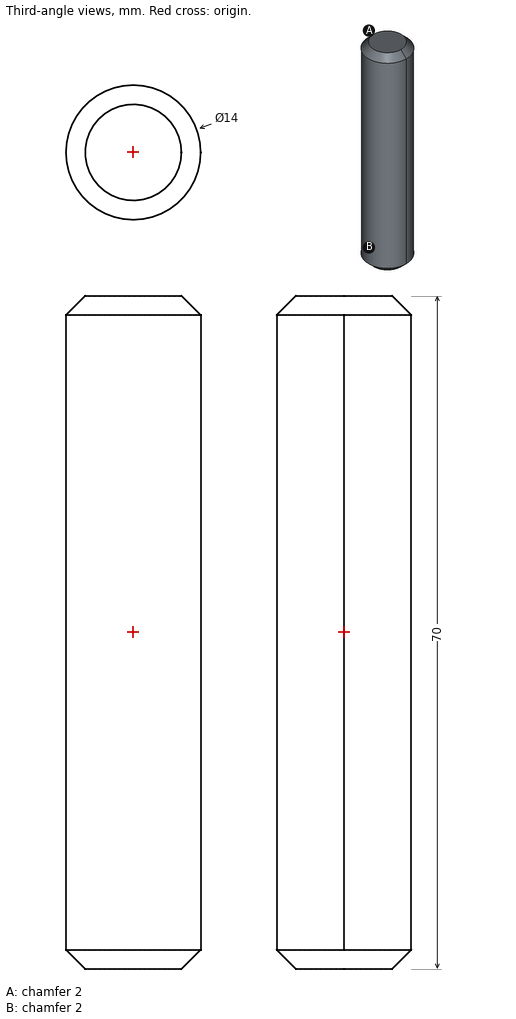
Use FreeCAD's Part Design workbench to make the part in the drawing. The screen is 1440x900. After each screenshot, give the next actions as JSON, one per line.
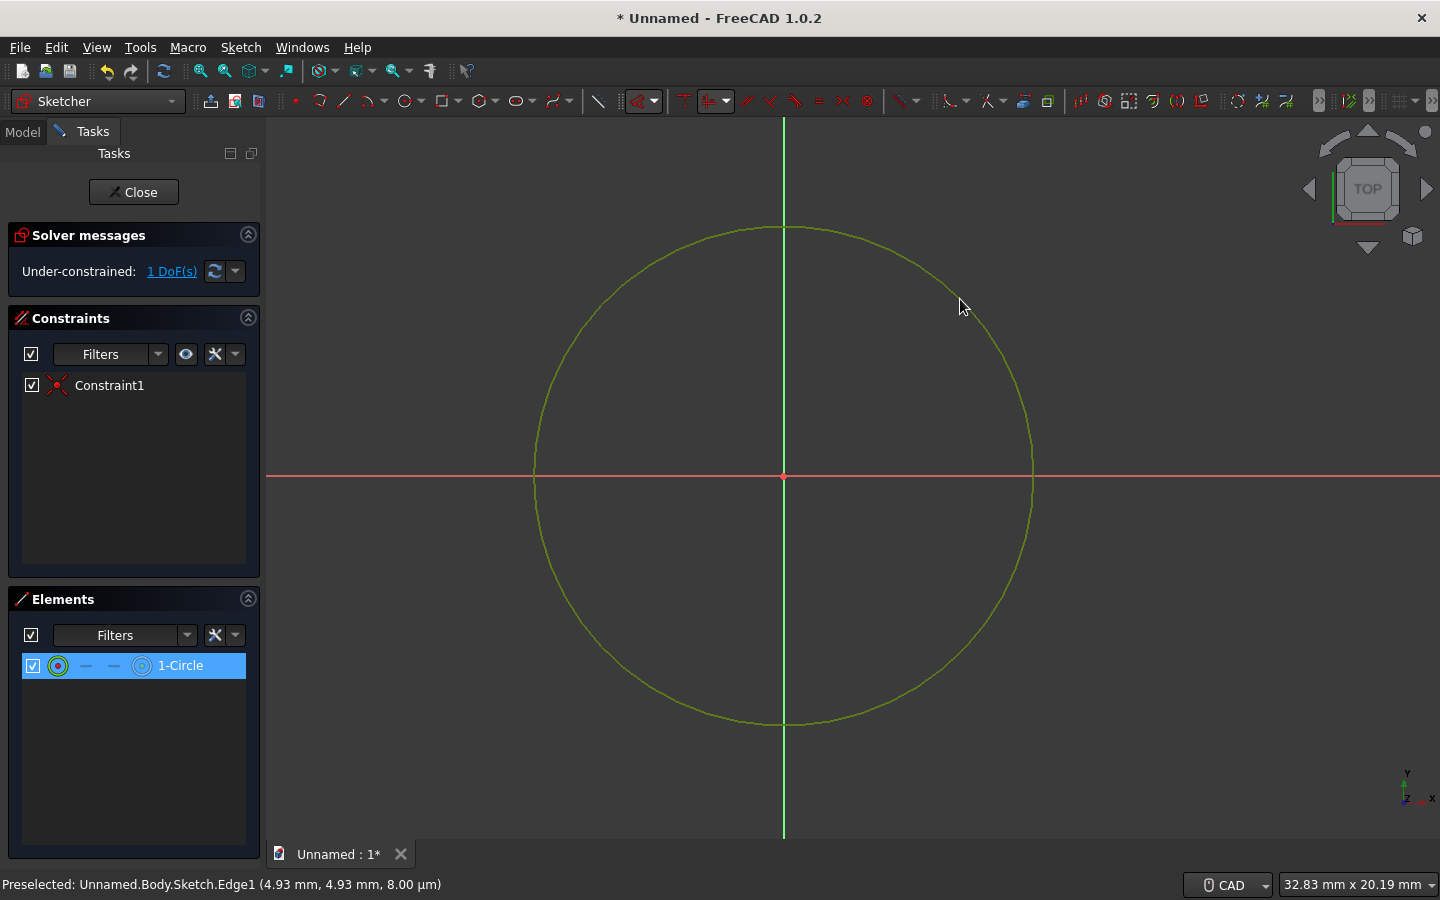
{"action": "key", "text": "k o"}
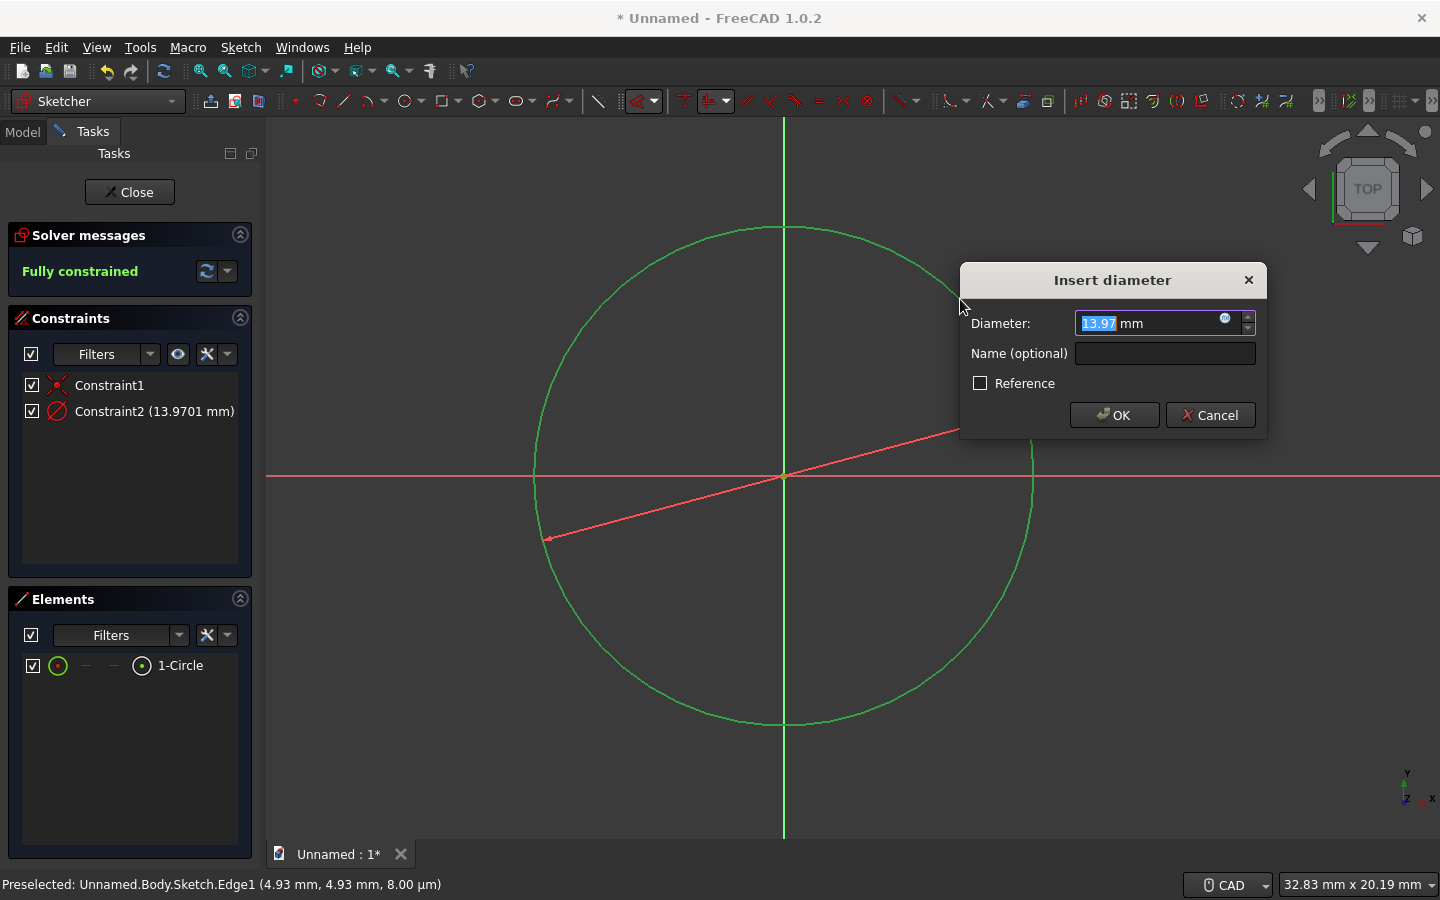
{"action": "type", "text": "14"}
{"action": "key", "text": "Return"}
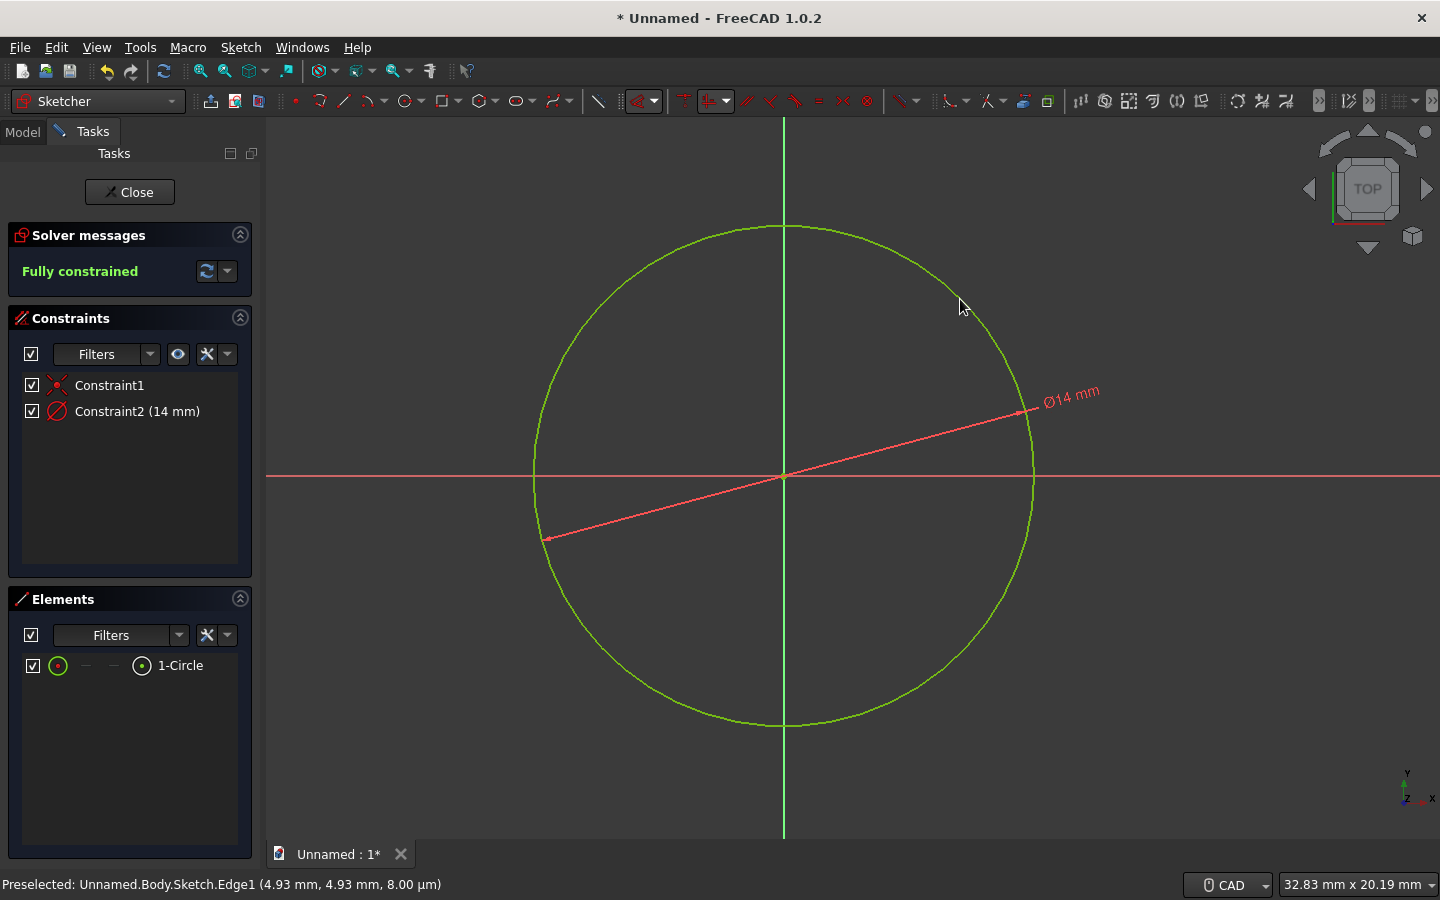
{"action": "left_click", "coordinate": [130, 192]}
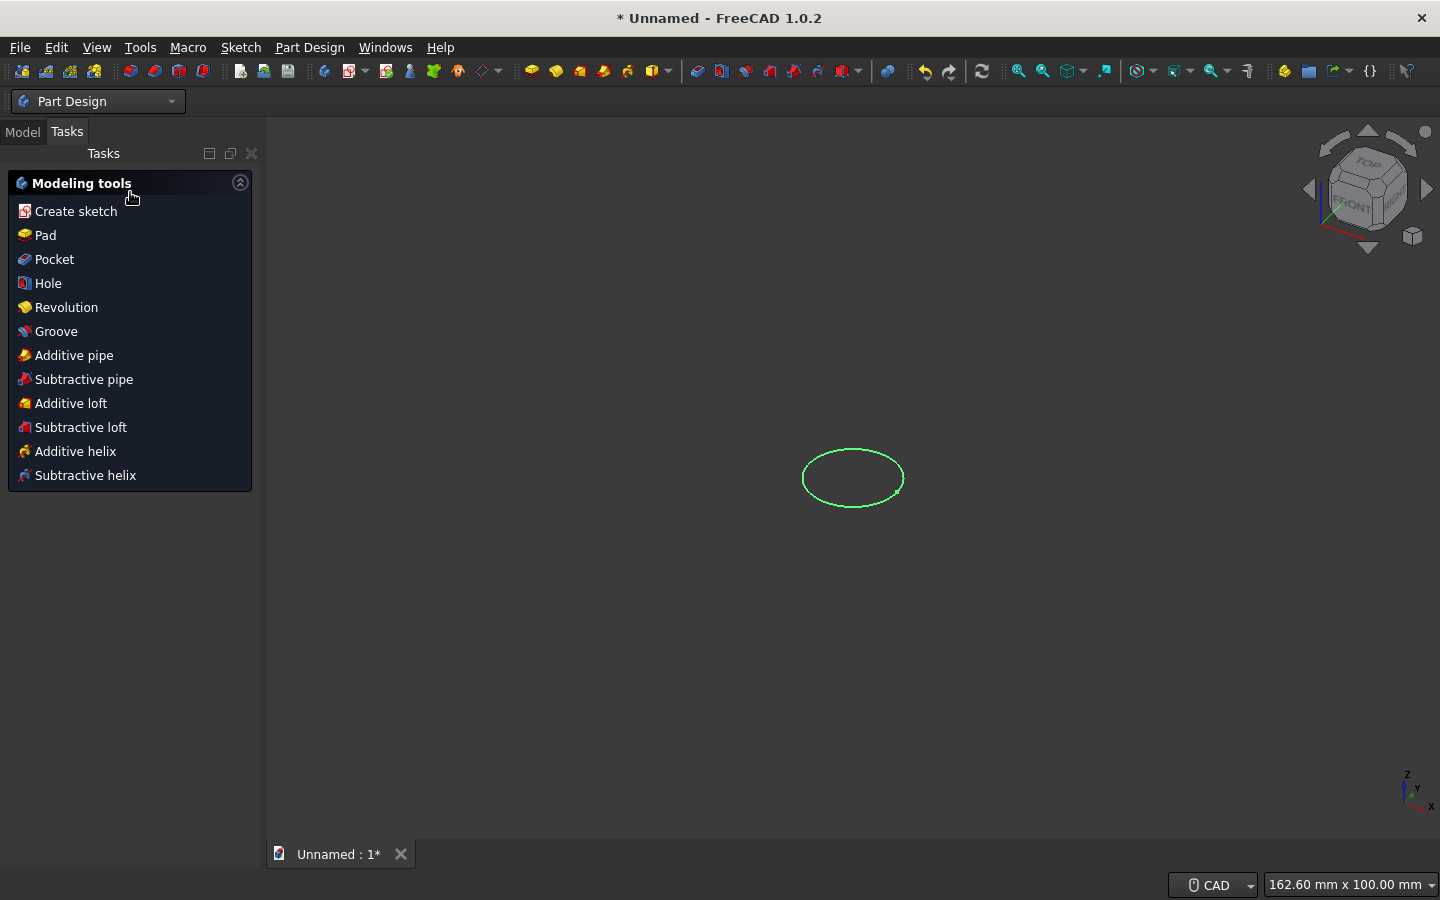
{"action": "left_click", "coordinate": [532, 72]}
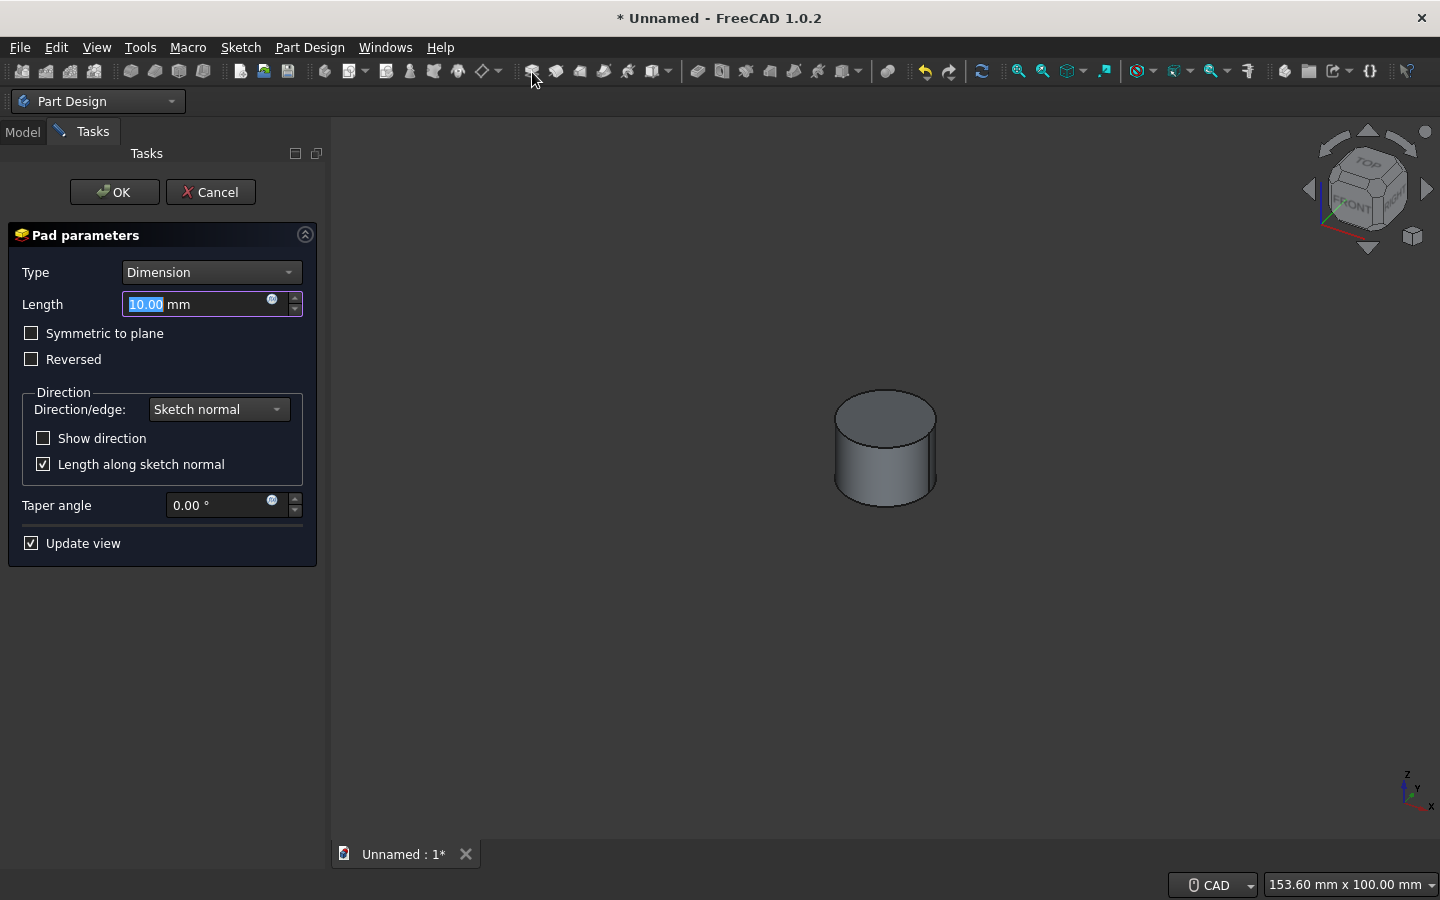
{"action": "type", "text": "70"}
{"action": "key", "text": "Tab"}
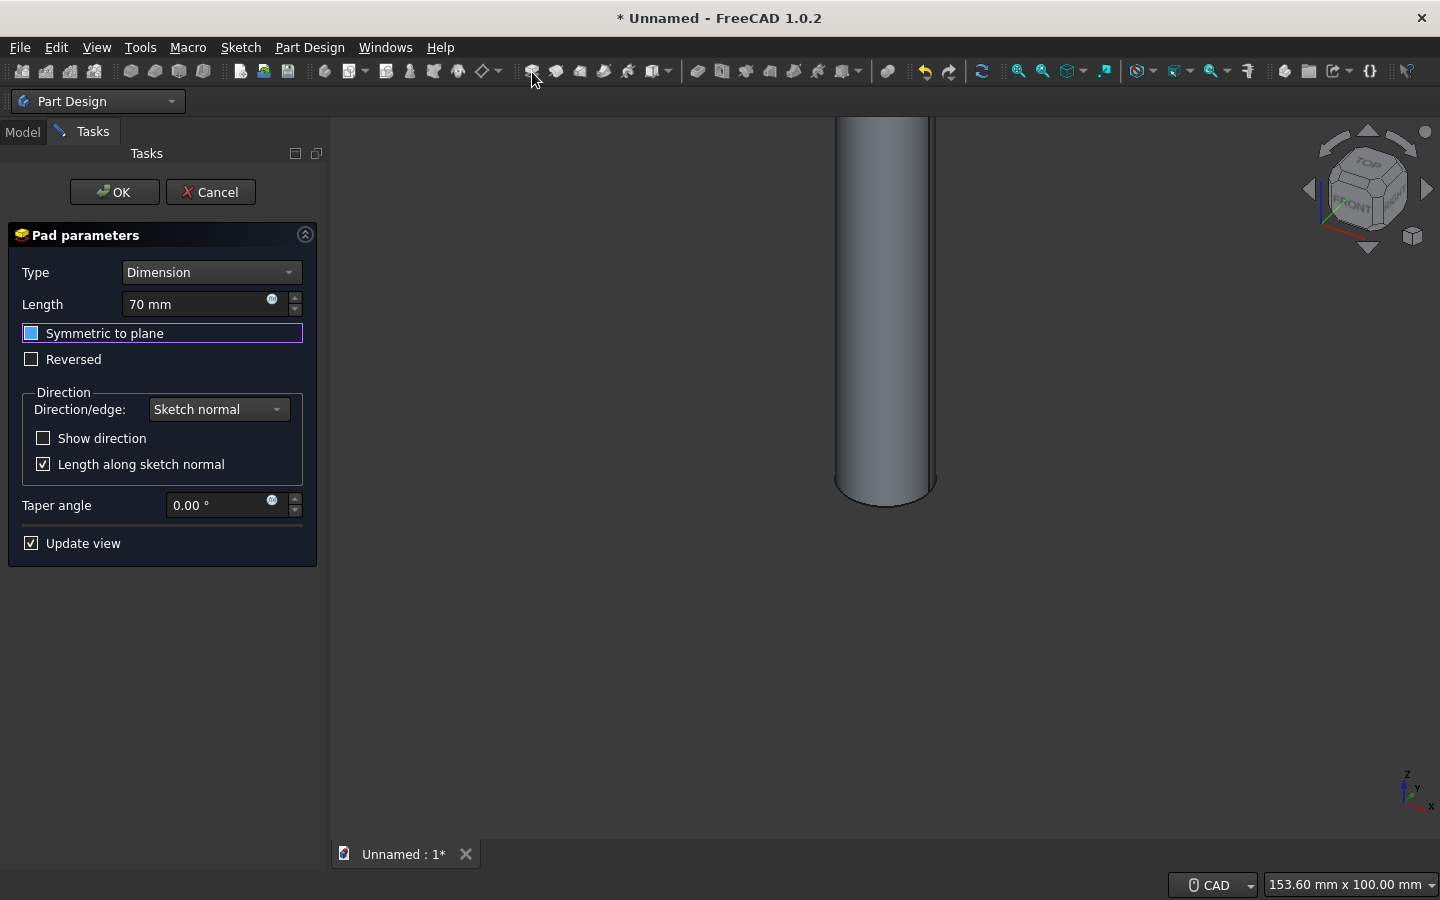
{"action": "left_click", "coordinate": [30, 333]}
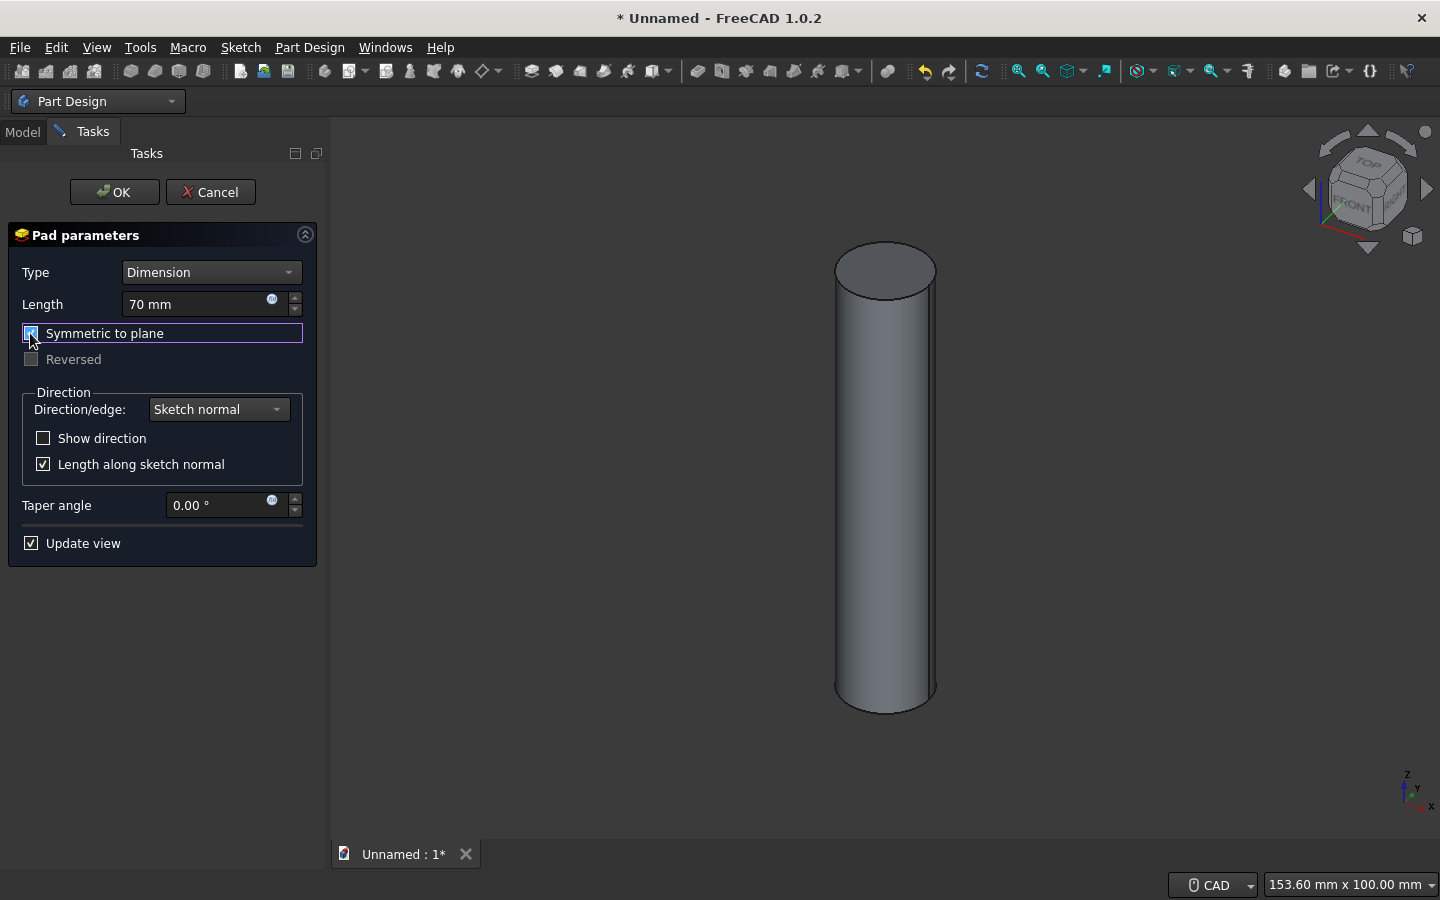
{"action": "left_click", "coordinate": [115, 192]}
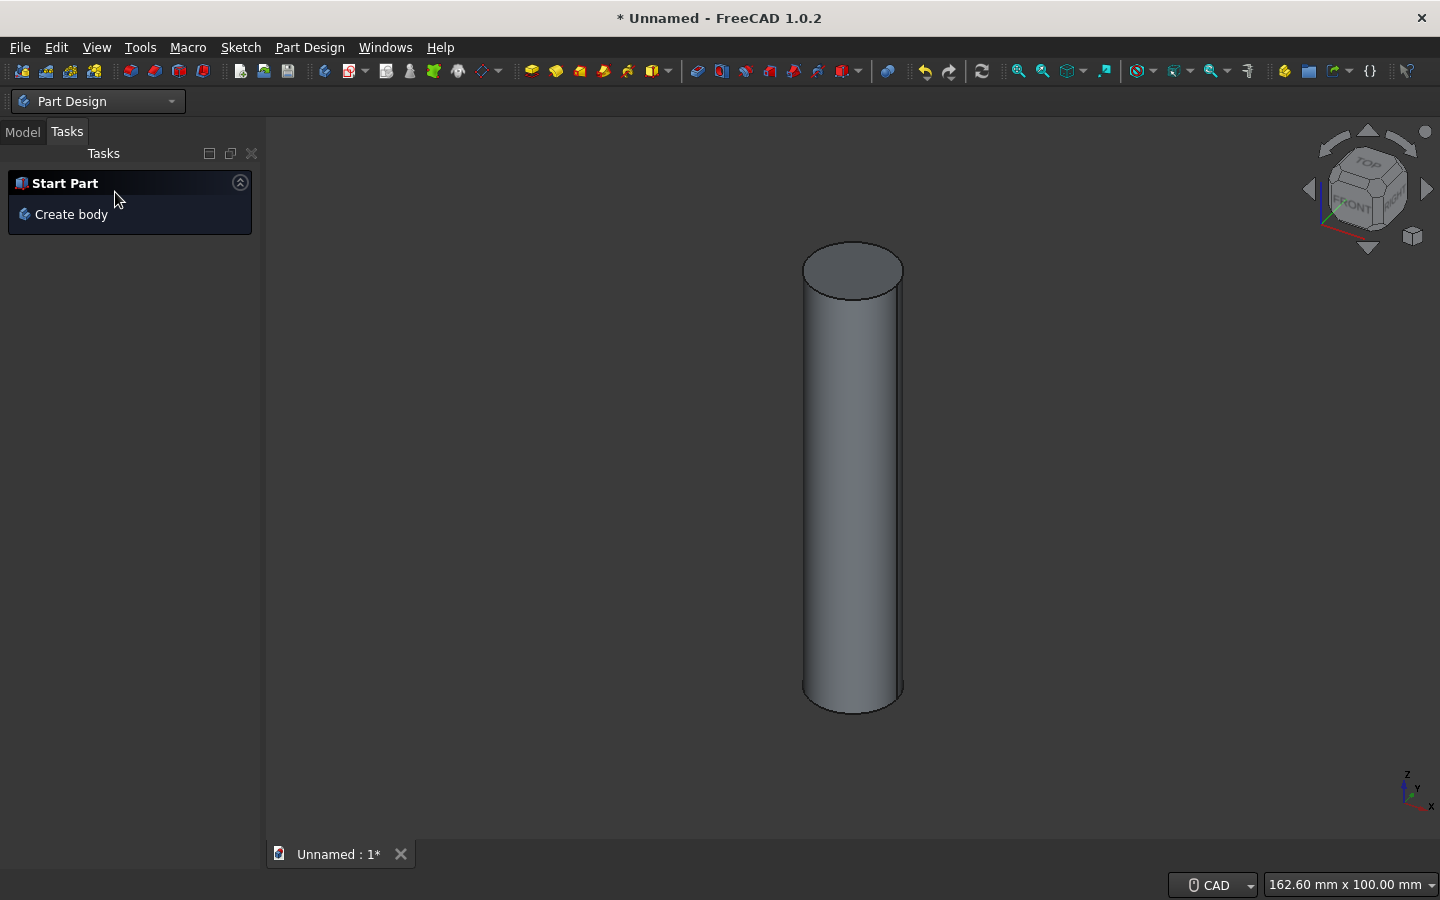
{"action": "left_click", "coordinate": [809, 256]}